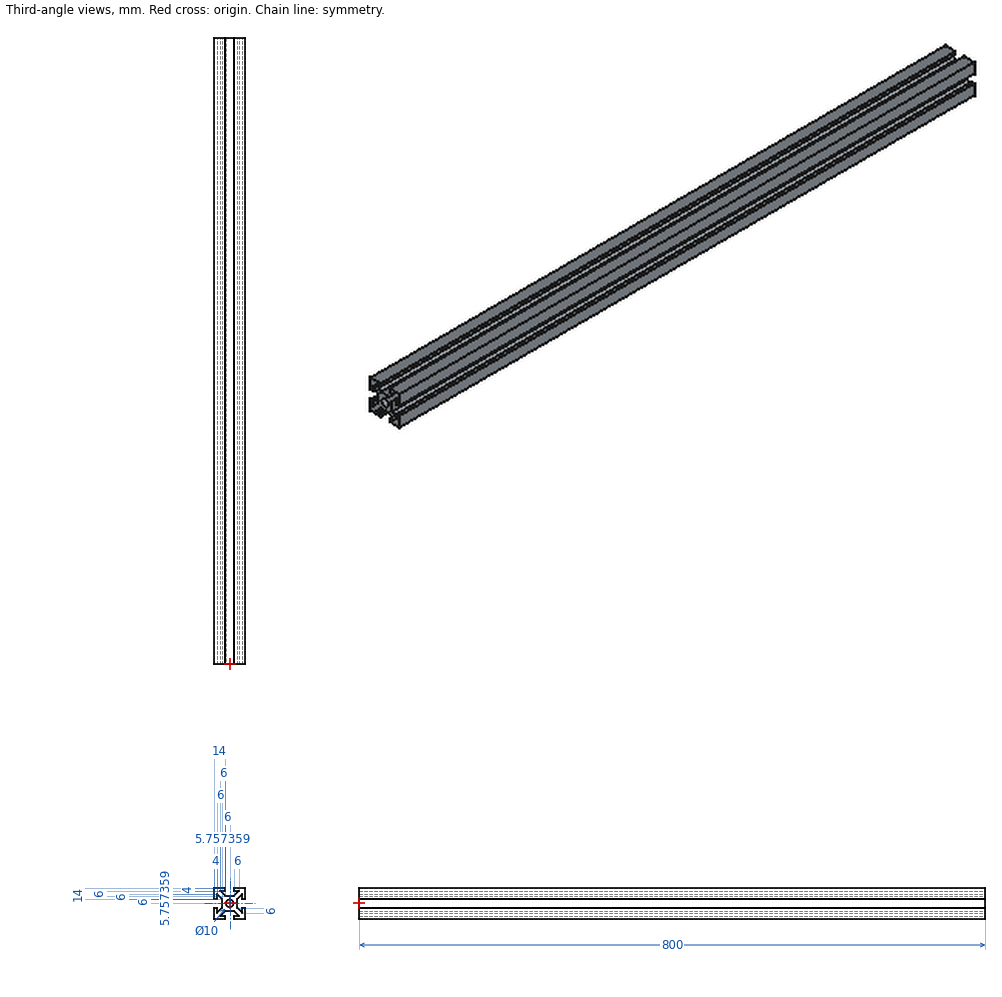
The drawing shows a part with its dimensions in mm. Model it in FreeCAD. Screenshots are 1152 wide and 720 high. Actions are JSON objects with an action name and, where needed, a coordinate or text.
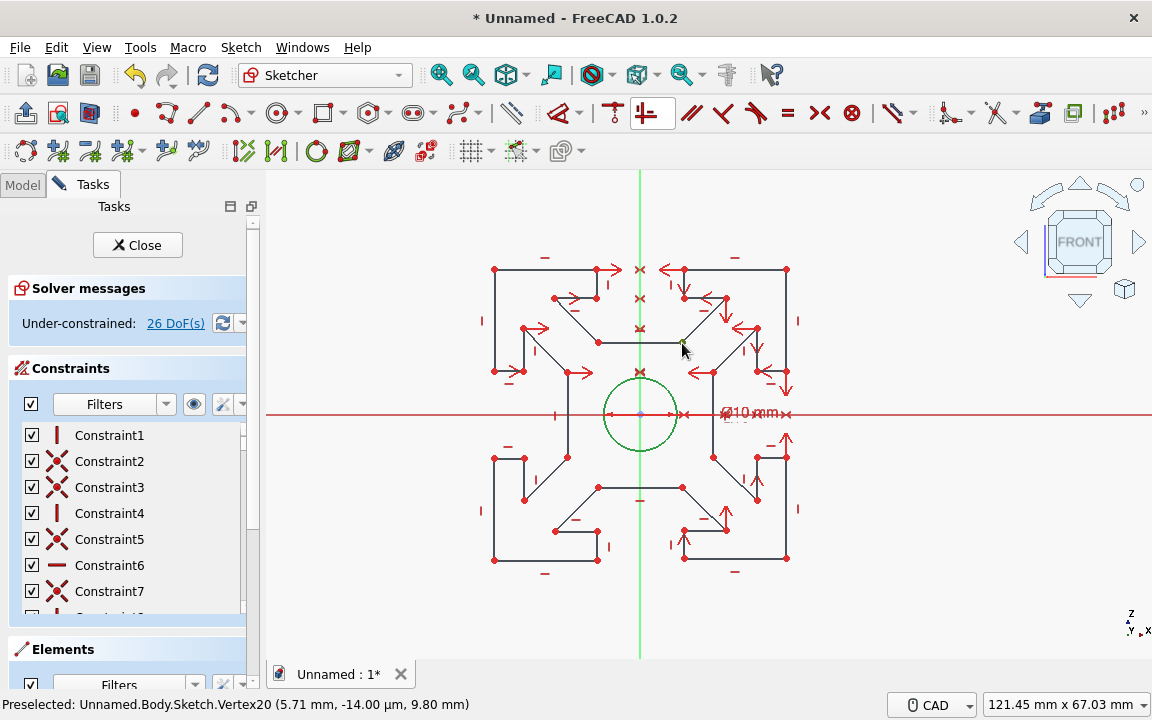
{"action": "left_click", "coordinate": [682, 488]}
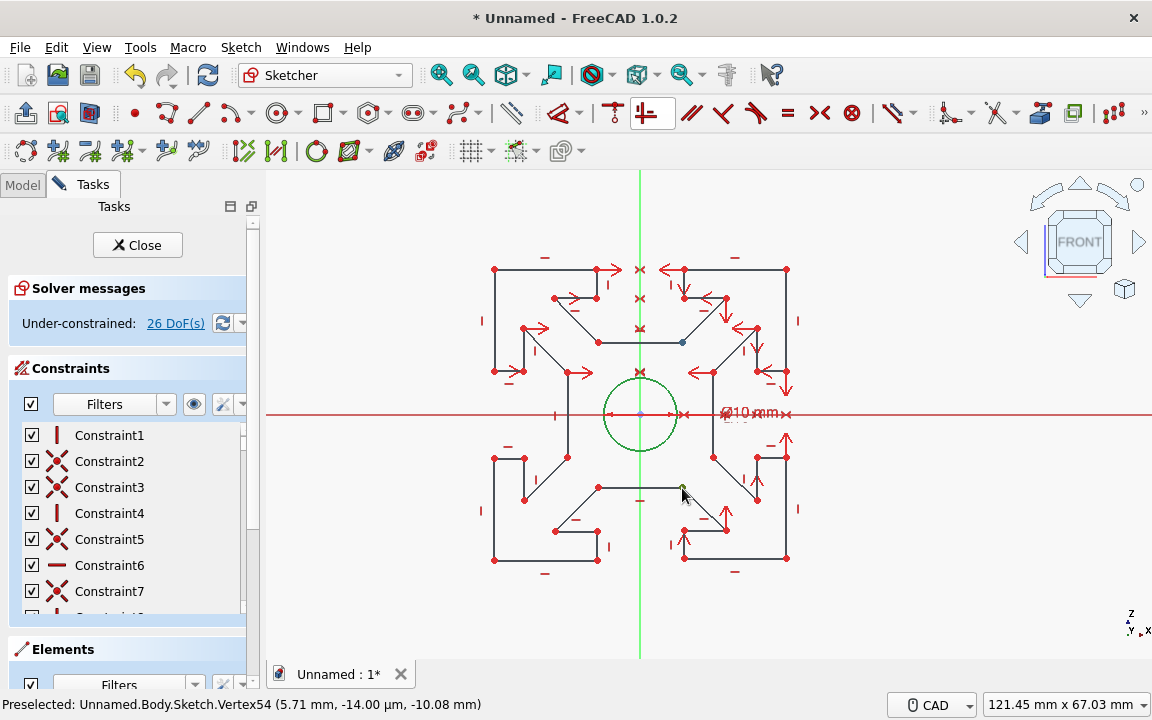
{"action": "left_click", "coordinate": [344, 414]}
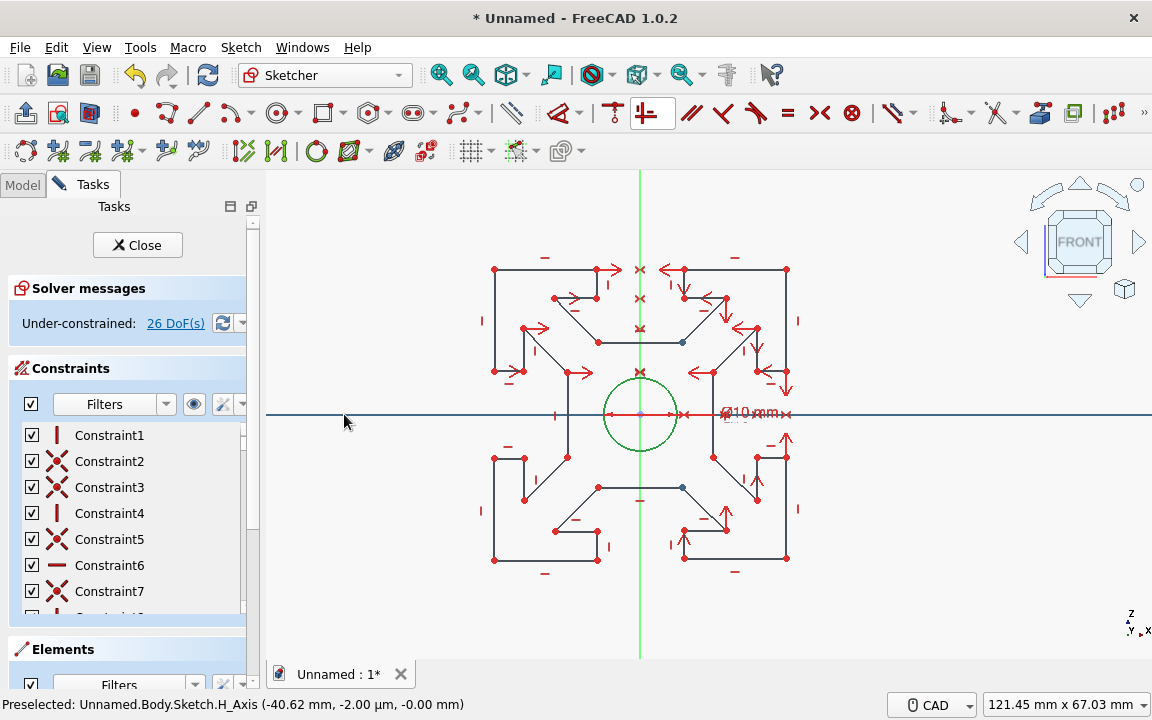
{"action": "key", "text": "s"}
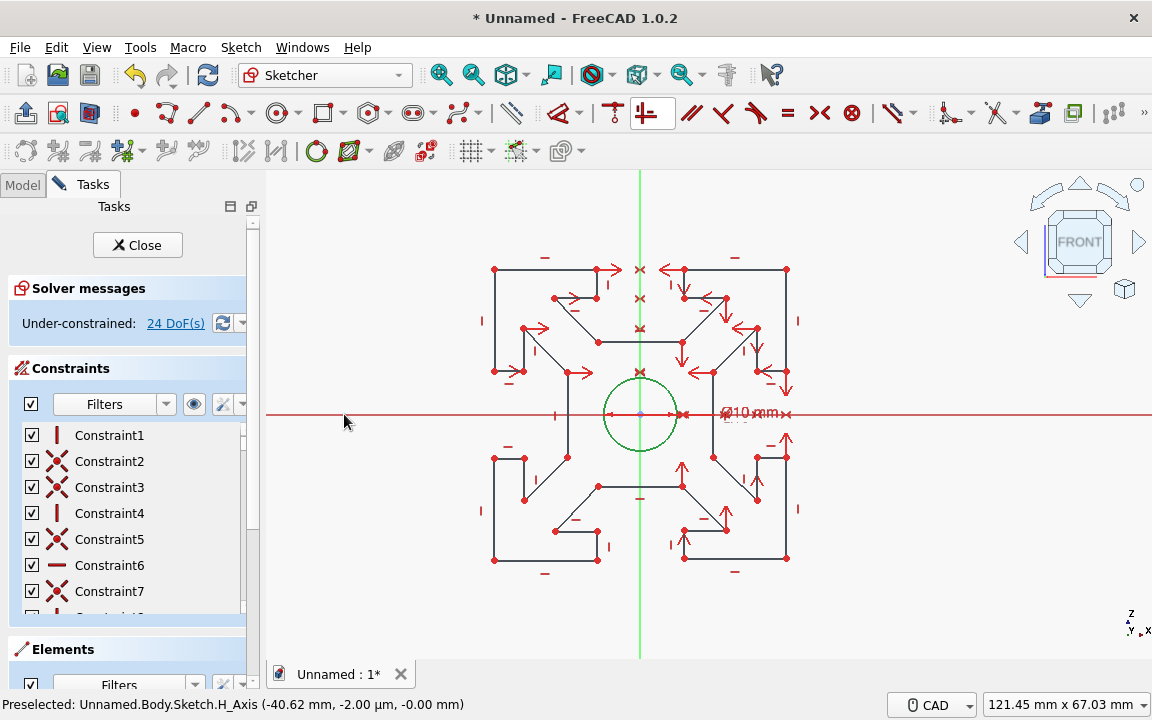
{"action": "left_click", "coordinate": [555, 298]}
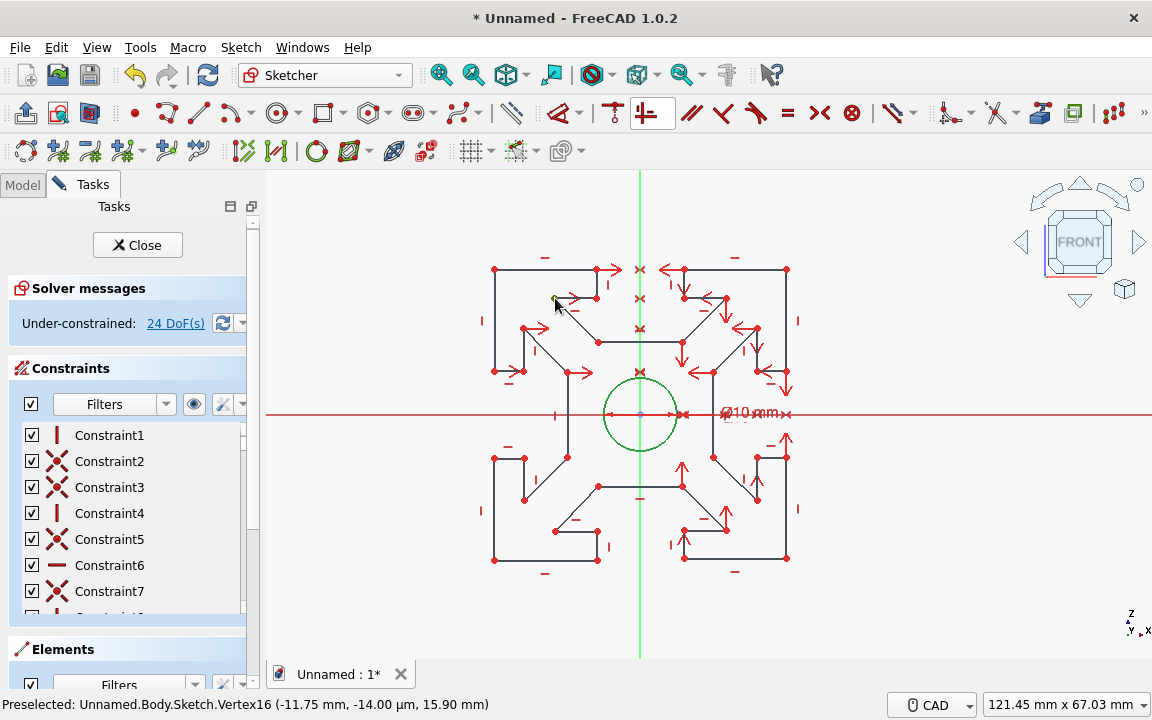
{"action": "left_click", "coordinate": [555, 532]}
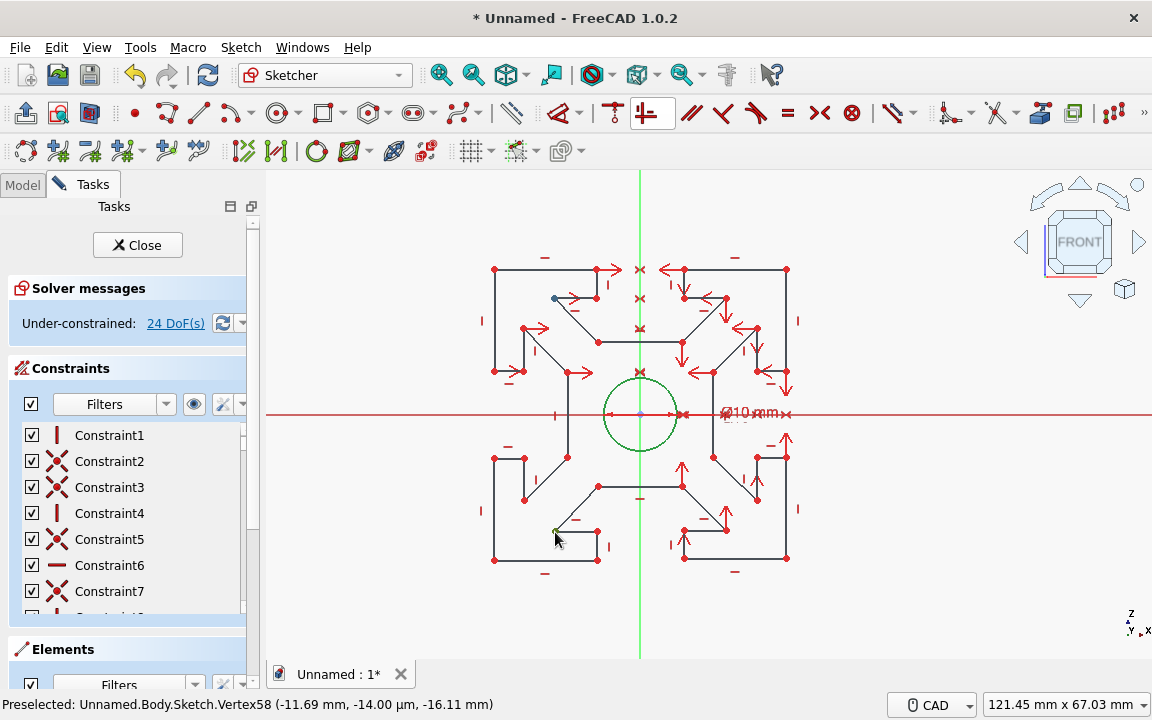
{"action": "left_click", "coordinate": [344, 414]}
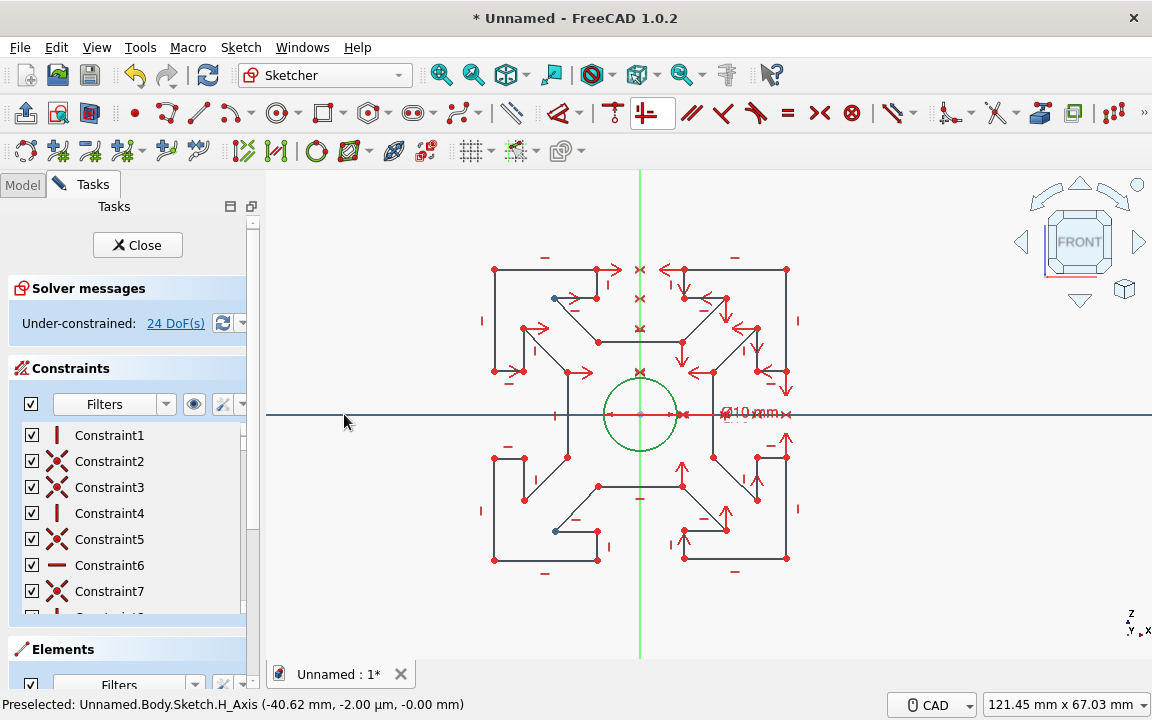
{"action": "left_click", "coordinate": [820, 114]}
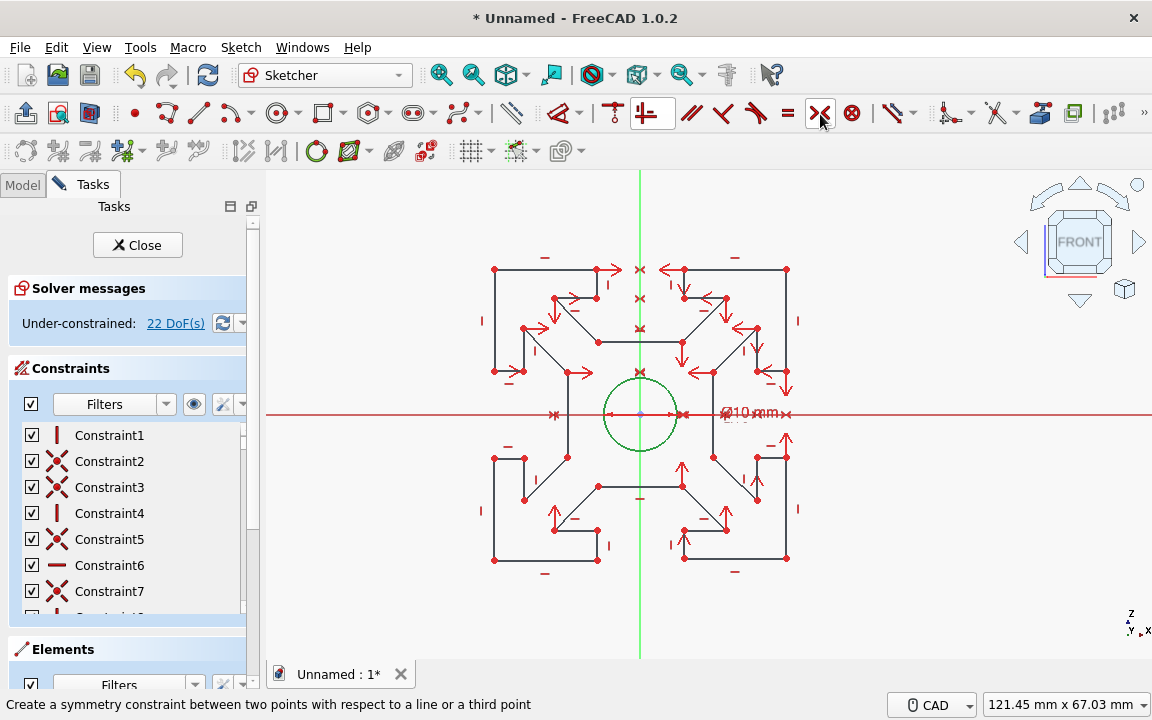
{"action": "left_click", "coordinate": [597, 270]}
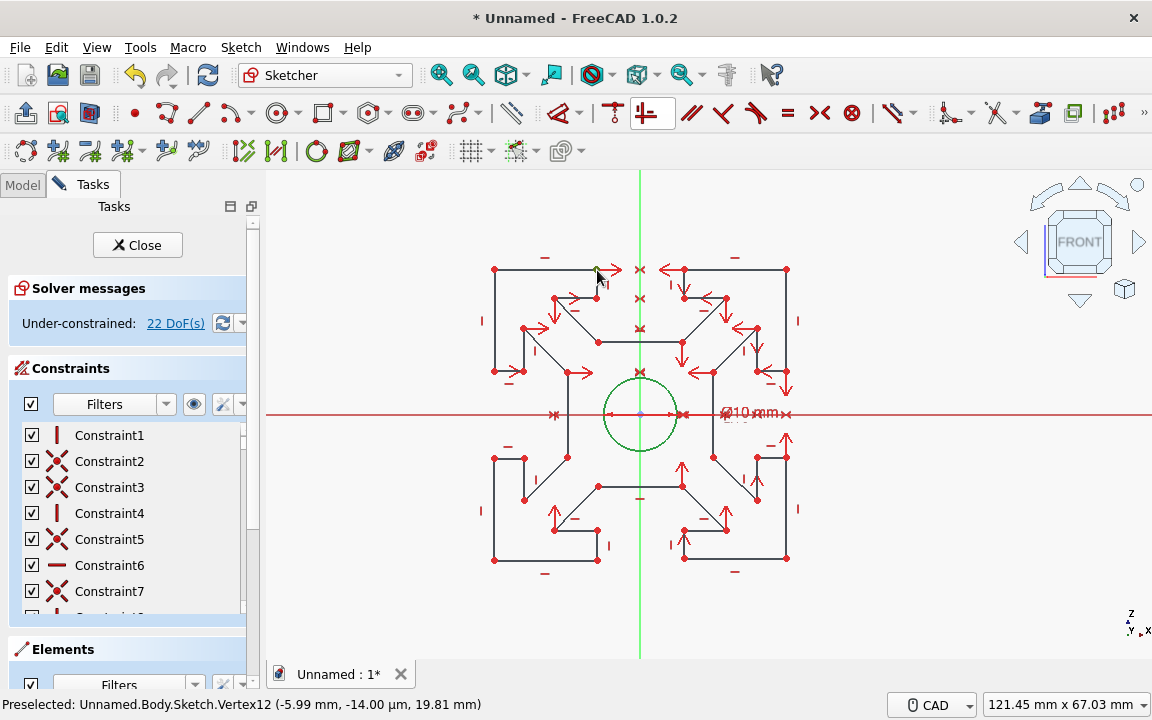
{"action": "left_click", "coordinate": [597, 561]}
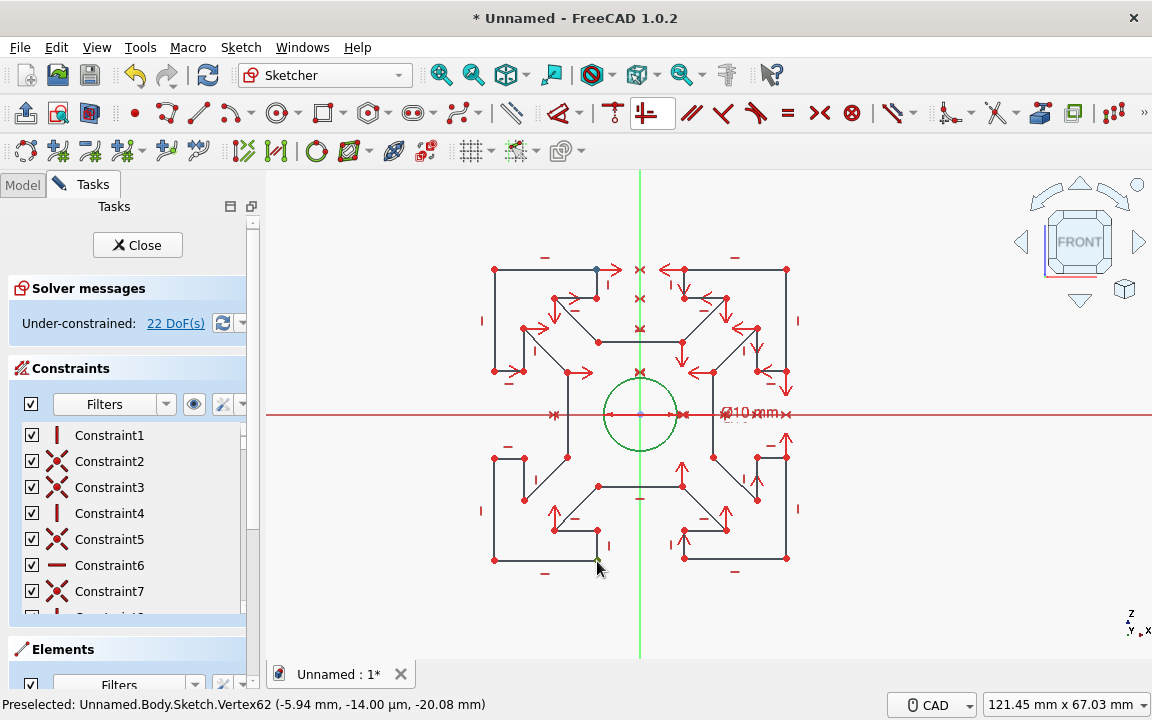
{"action": "left_click", "coordinate": [344, 414]}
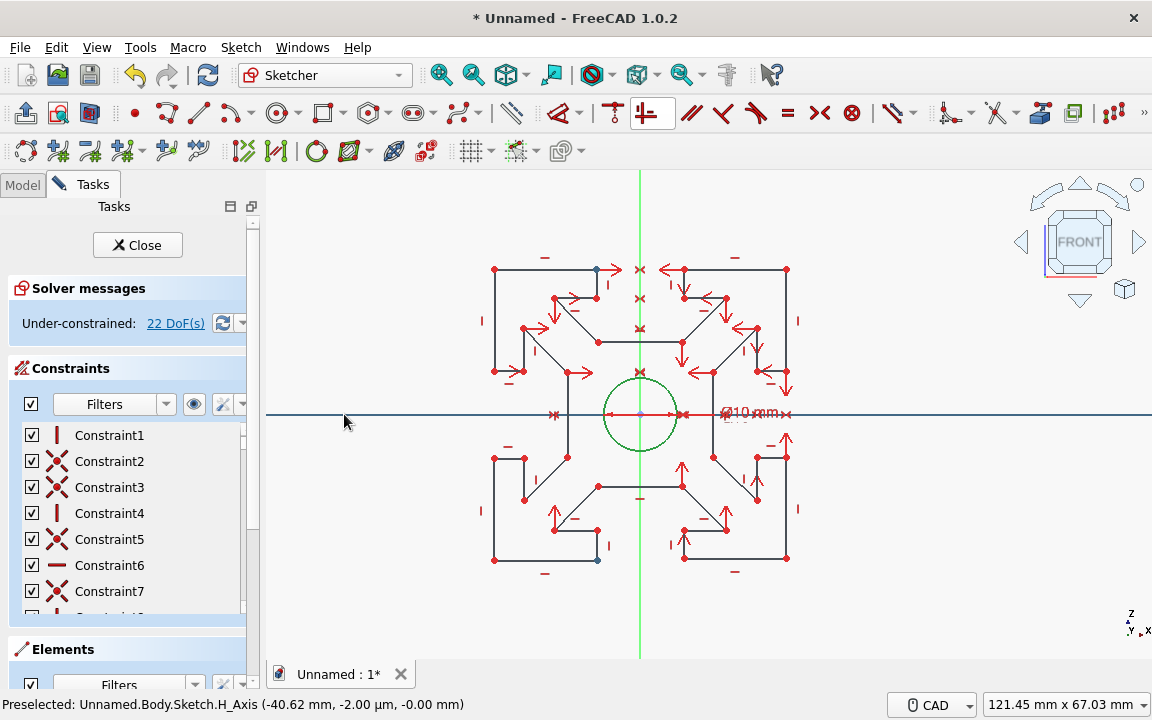
{"action": "left_click", "coordinate": [820, 114]}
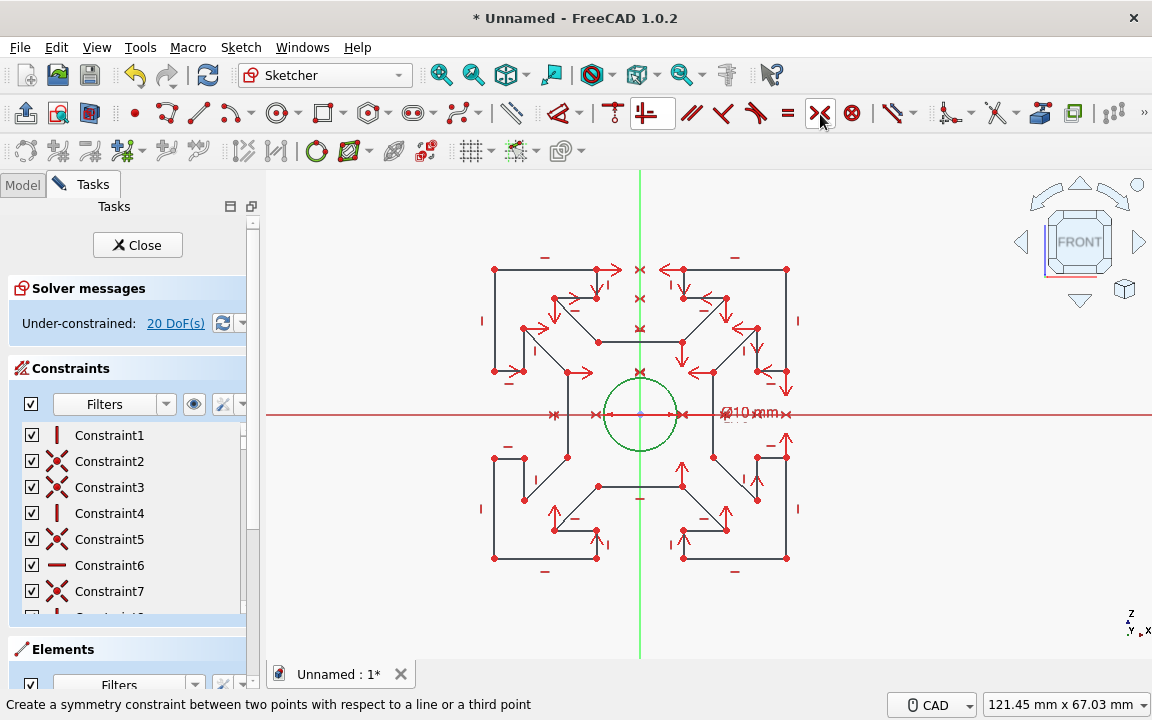
{"action": "left_click", "coordinate": [495, 371]}